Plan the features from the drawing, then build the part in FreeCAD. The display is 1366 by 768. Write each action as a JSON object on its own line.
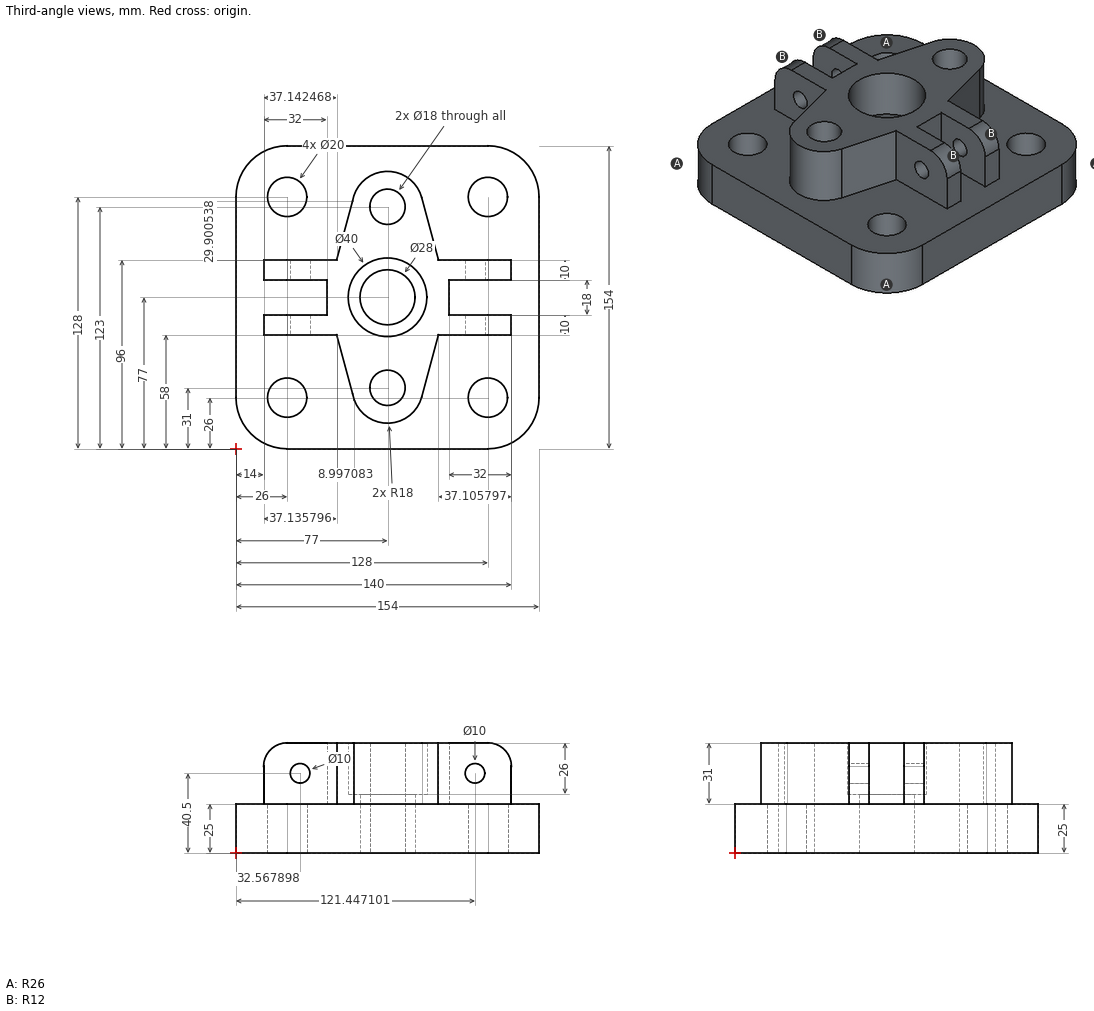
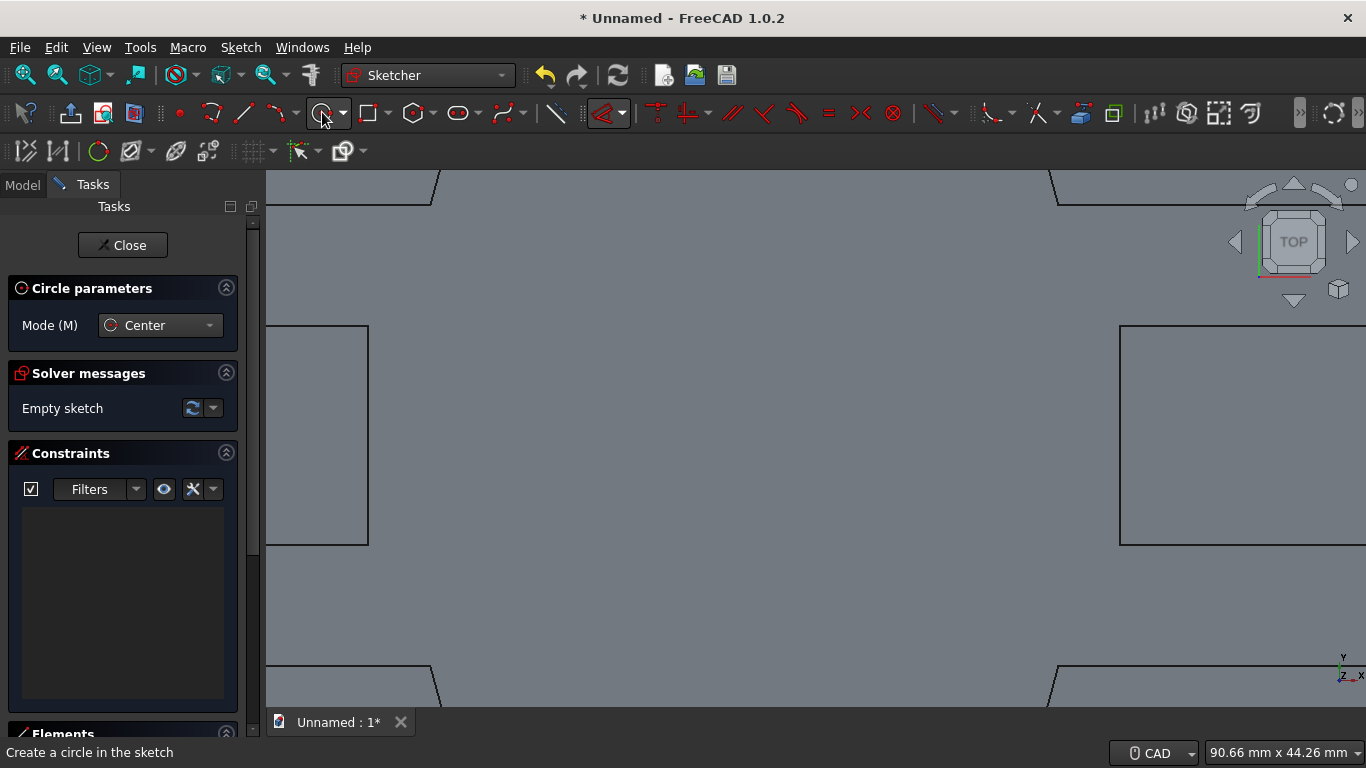
{"action": "left_click", "coordinate": [744, 436]}
{"action": "left_click", "coordinate": [864, 316]}
{"action": "key", "text": "Escape"}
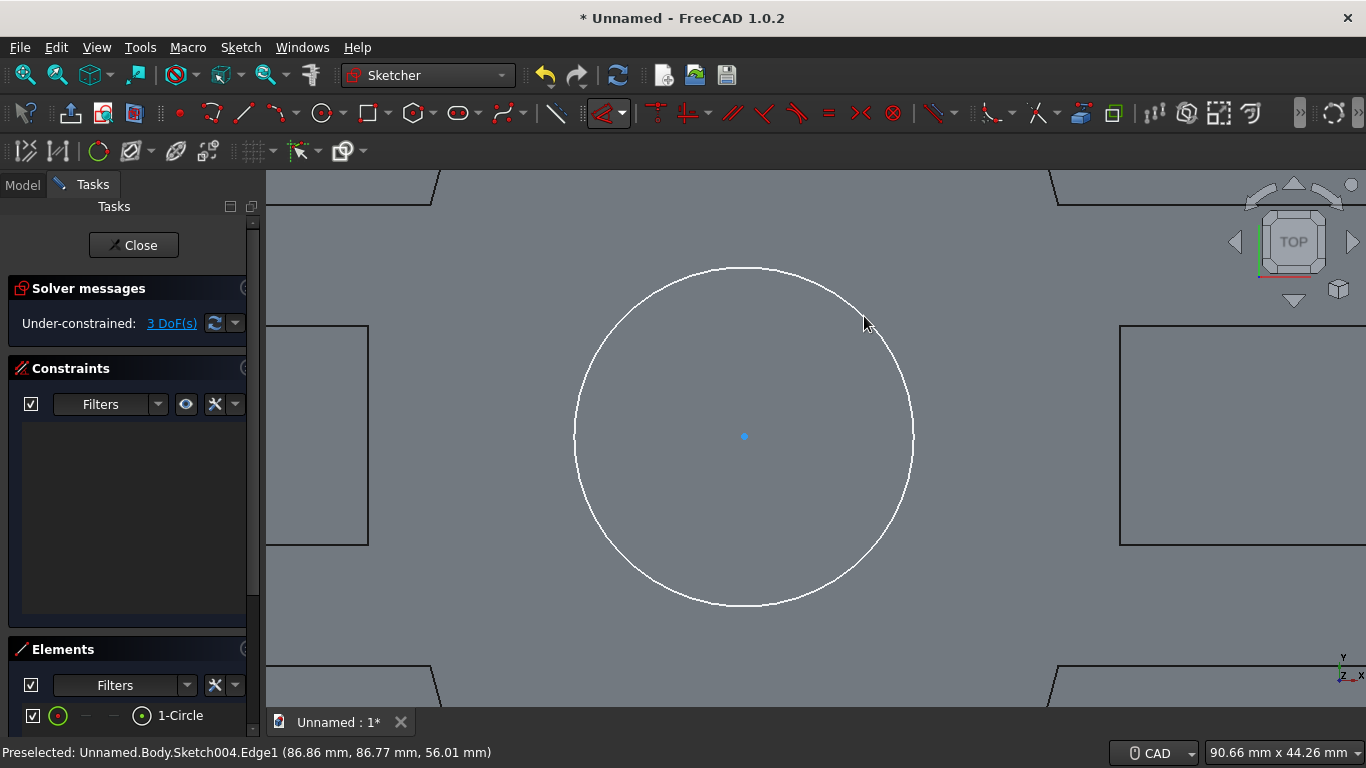
{"action": "left_click", "coordinate": [864, 317]}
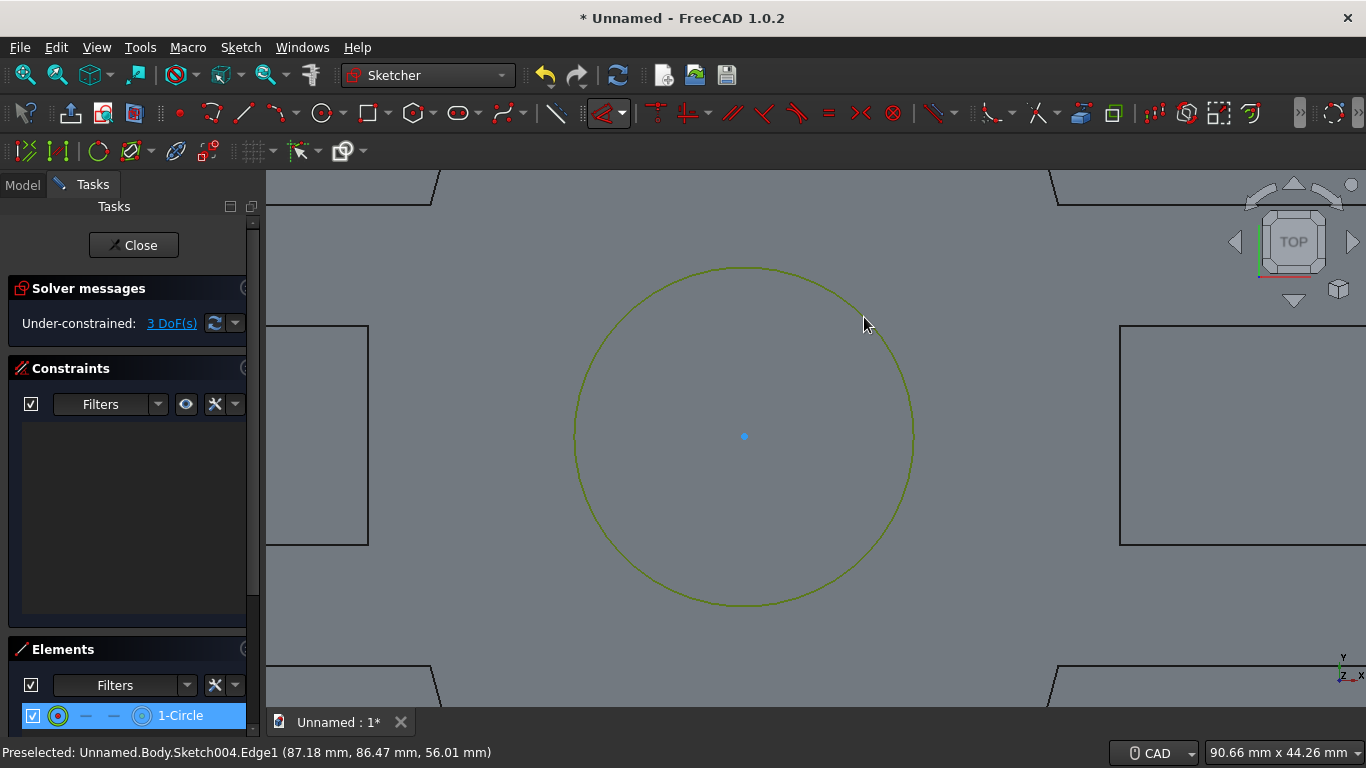
{"action": "left_click", "coordinate": [624, 114]}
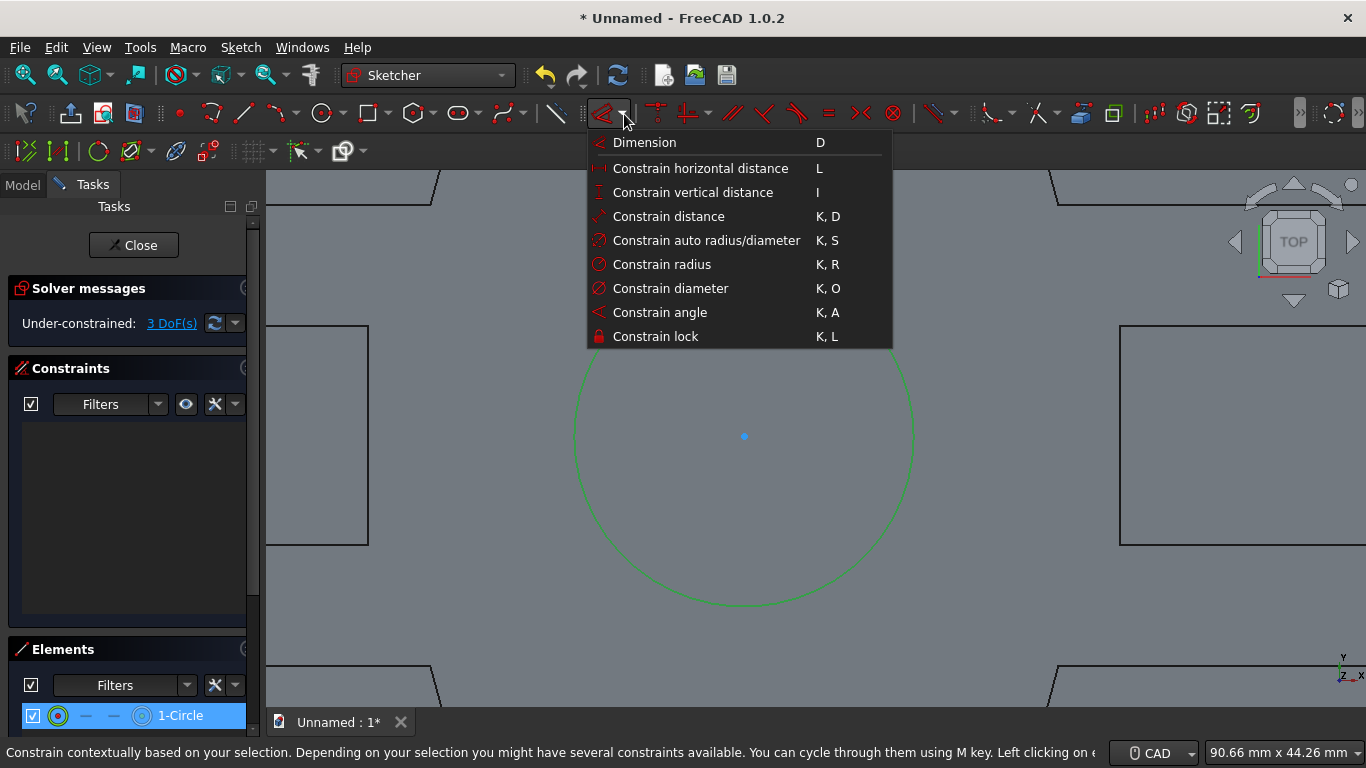
{"action": "left_click", "coordinate": [740, 288]}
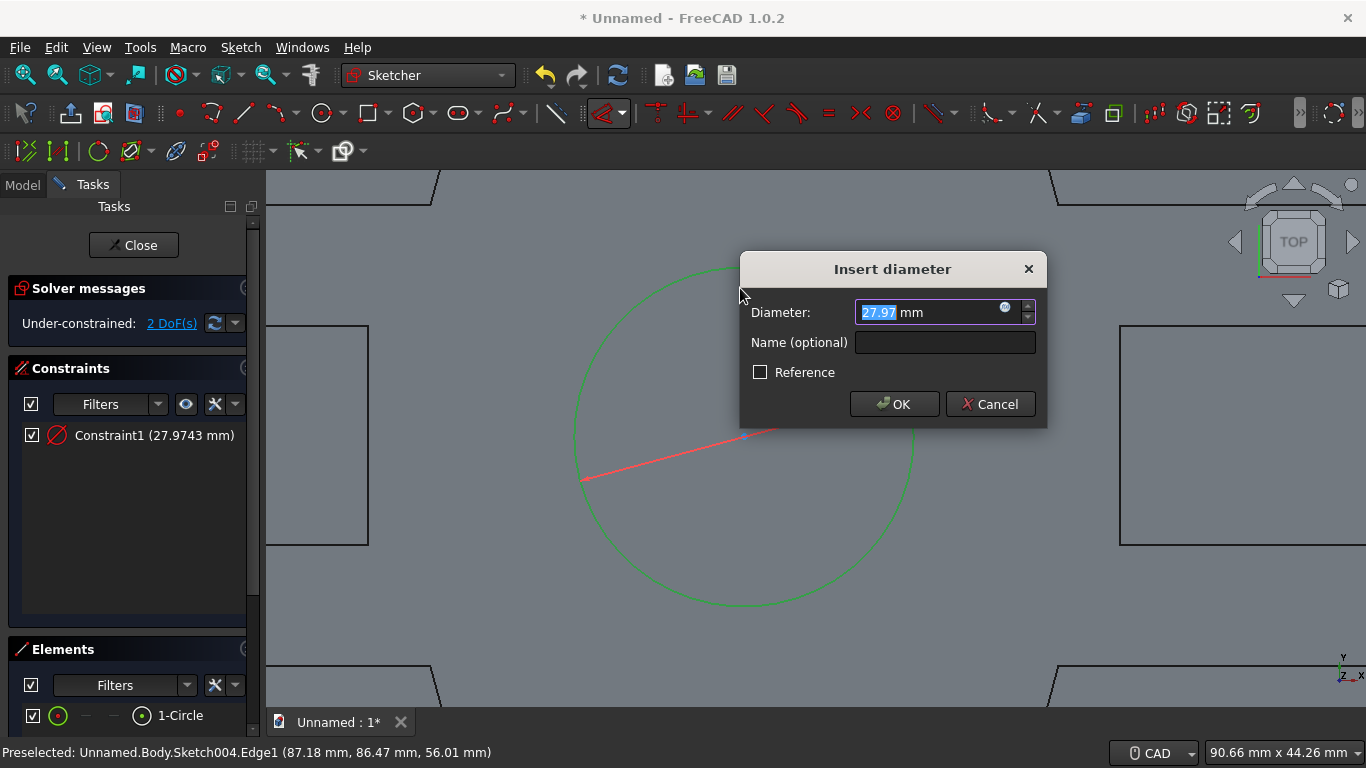
{"action": "type", "text": "28"}
{"action": "key", "text": "Return"}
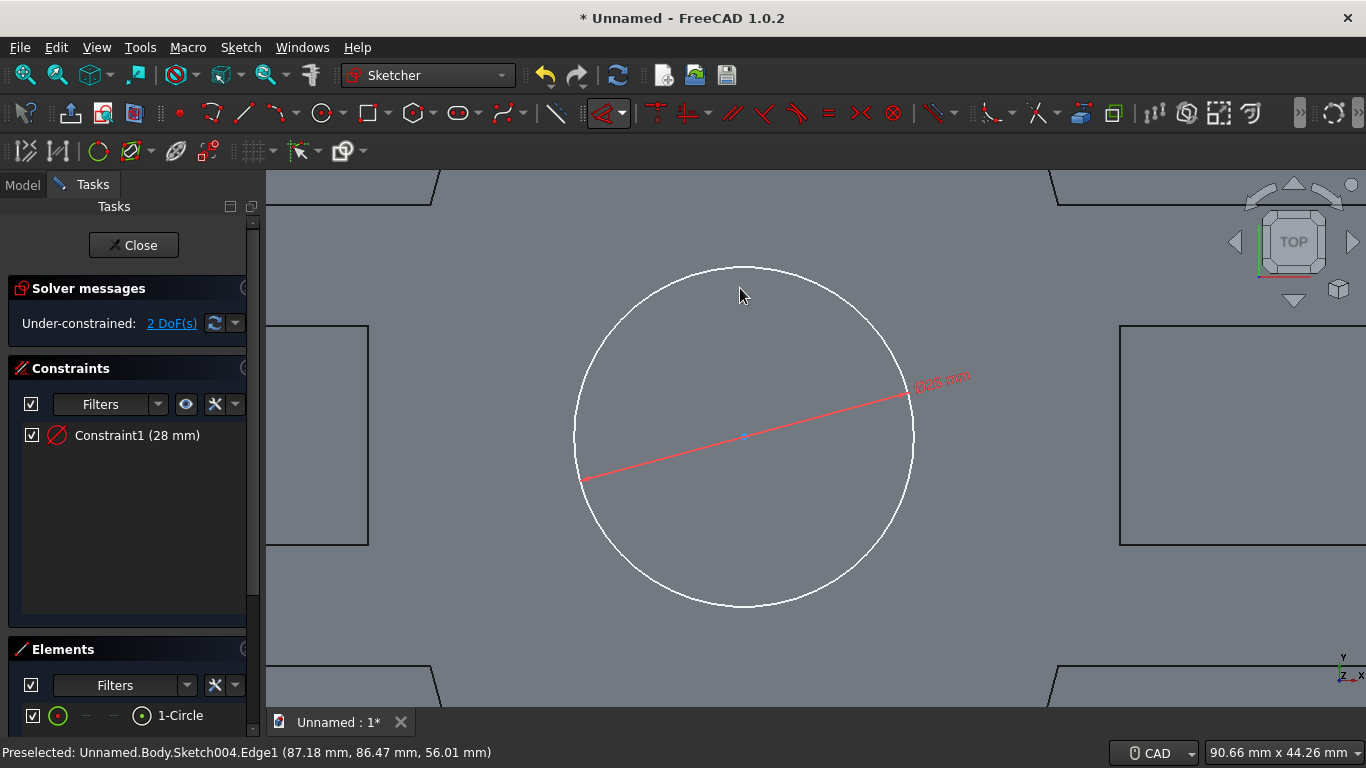
{"action": "left_click", "coordinate": [744, 437]}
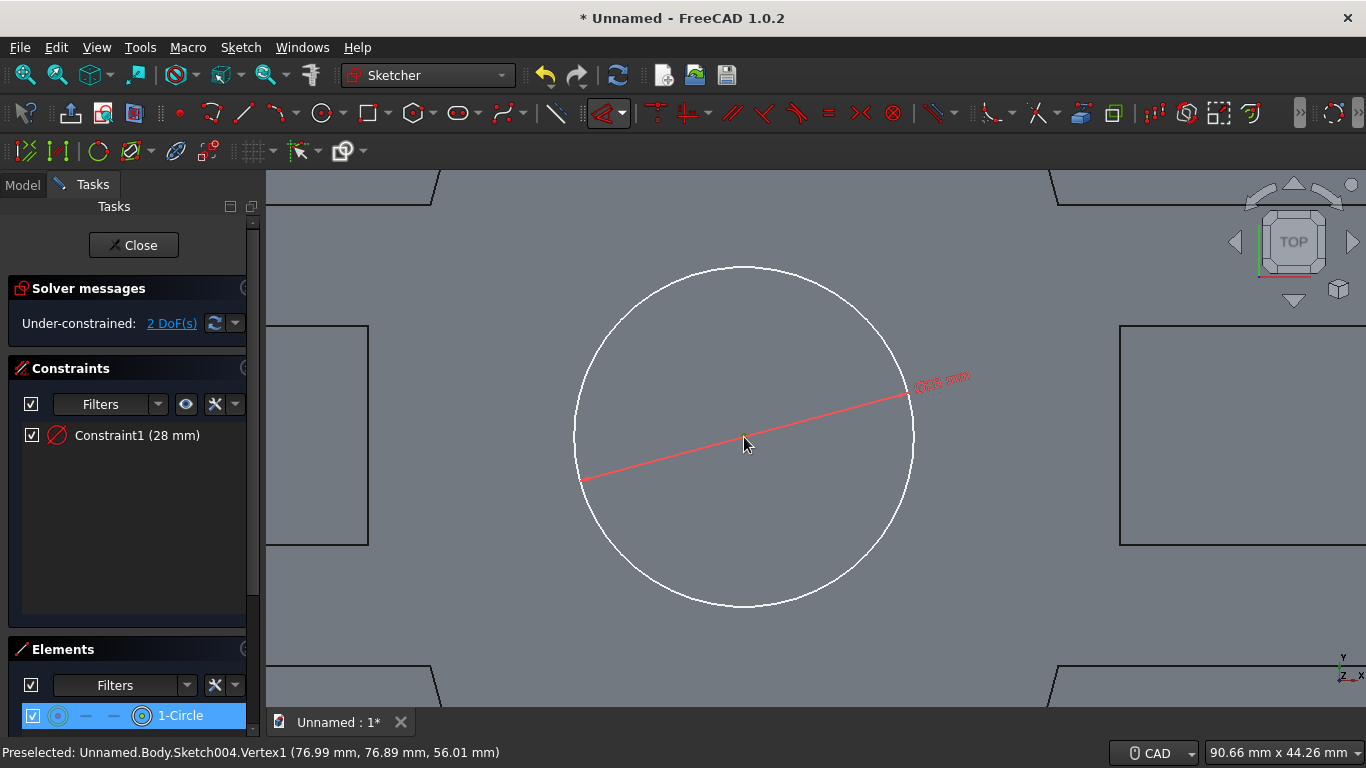
{"action": "key", "text": "l"}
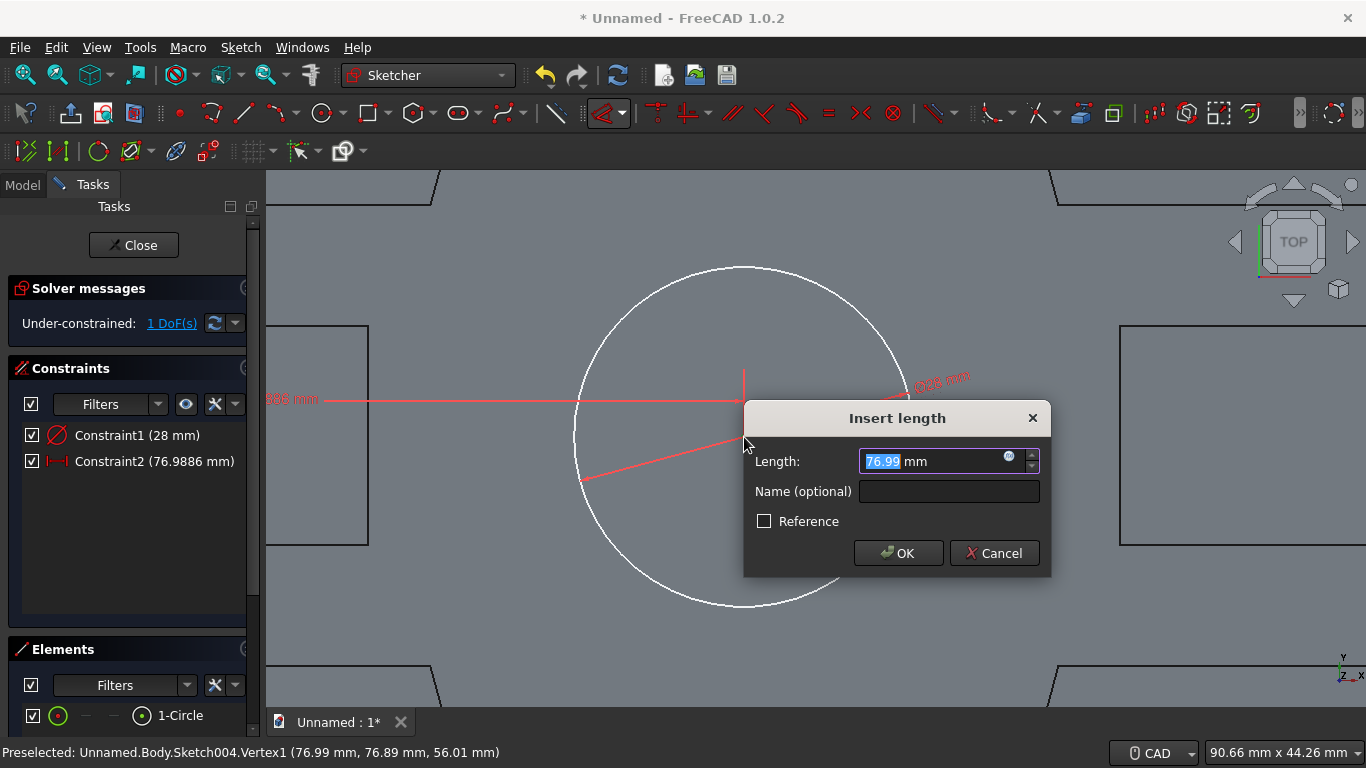
{"action": "type", "text": "77"}
{"action": "key", "text": "Return"}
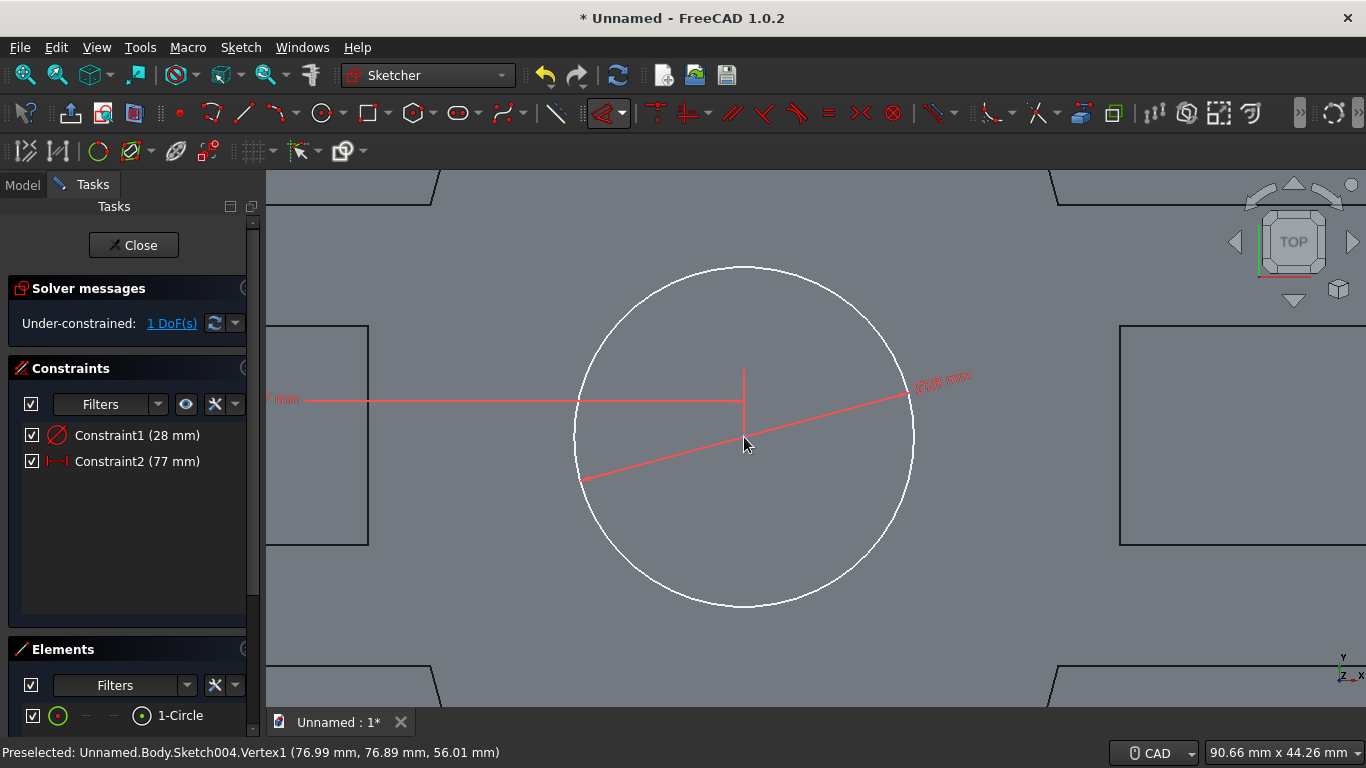
{"action": "left_click", "coordinate": [744, 437]}